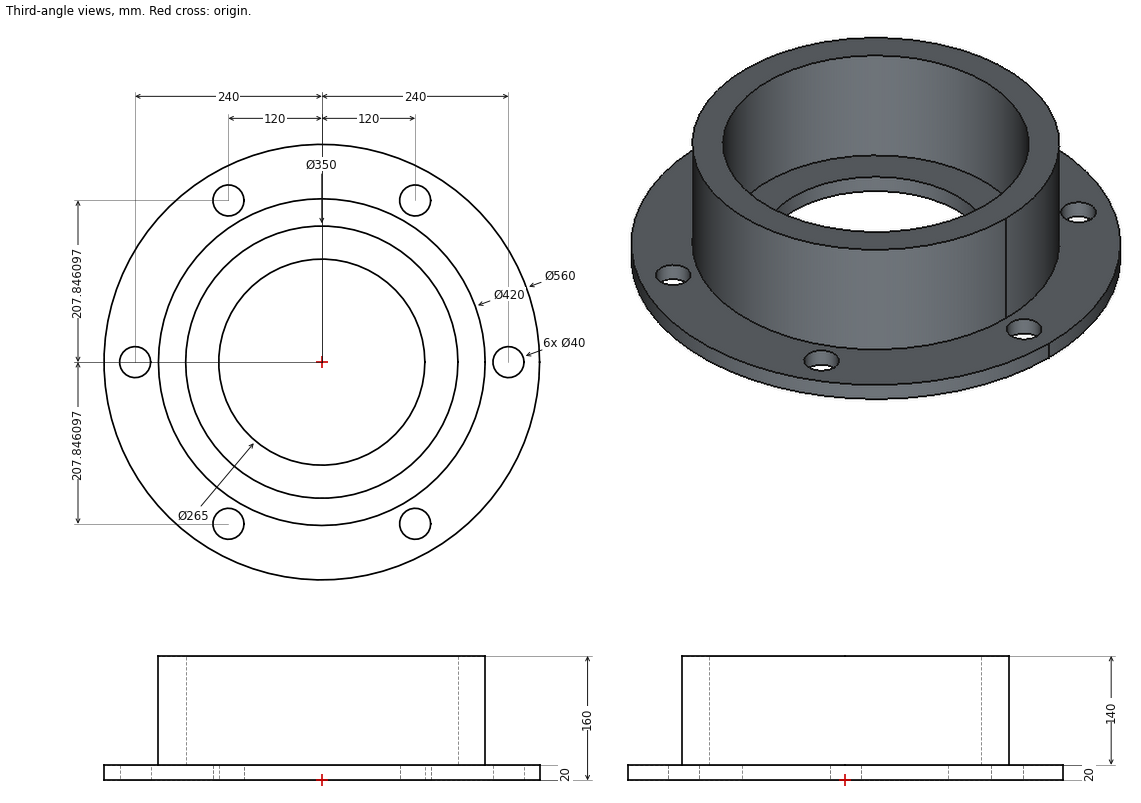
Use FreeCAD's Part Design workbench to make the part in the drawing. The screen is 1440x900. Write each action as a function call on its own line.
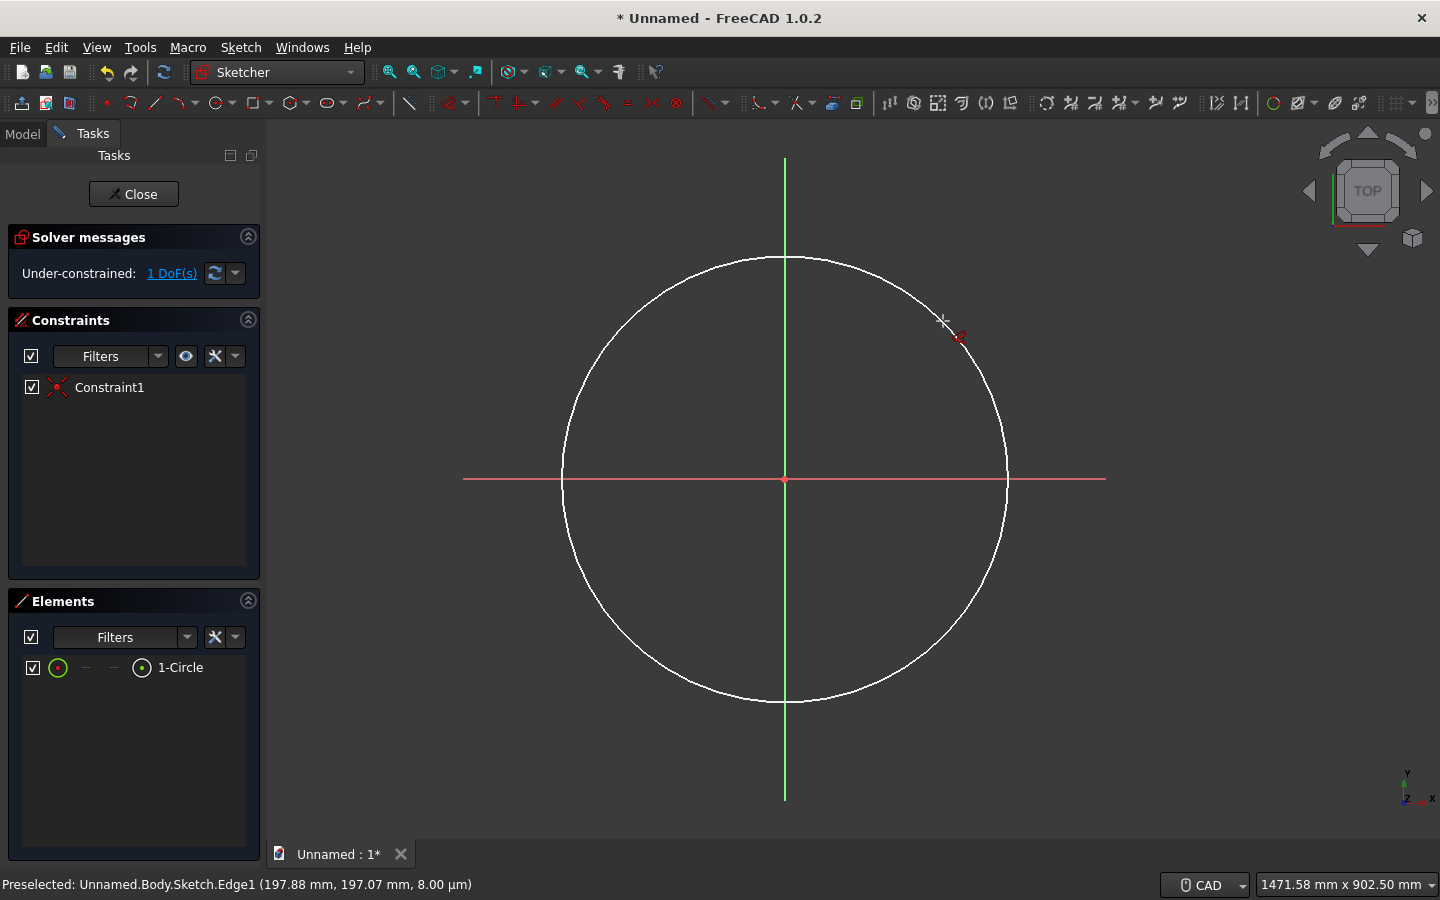
click(942, 321)
click(965, 298)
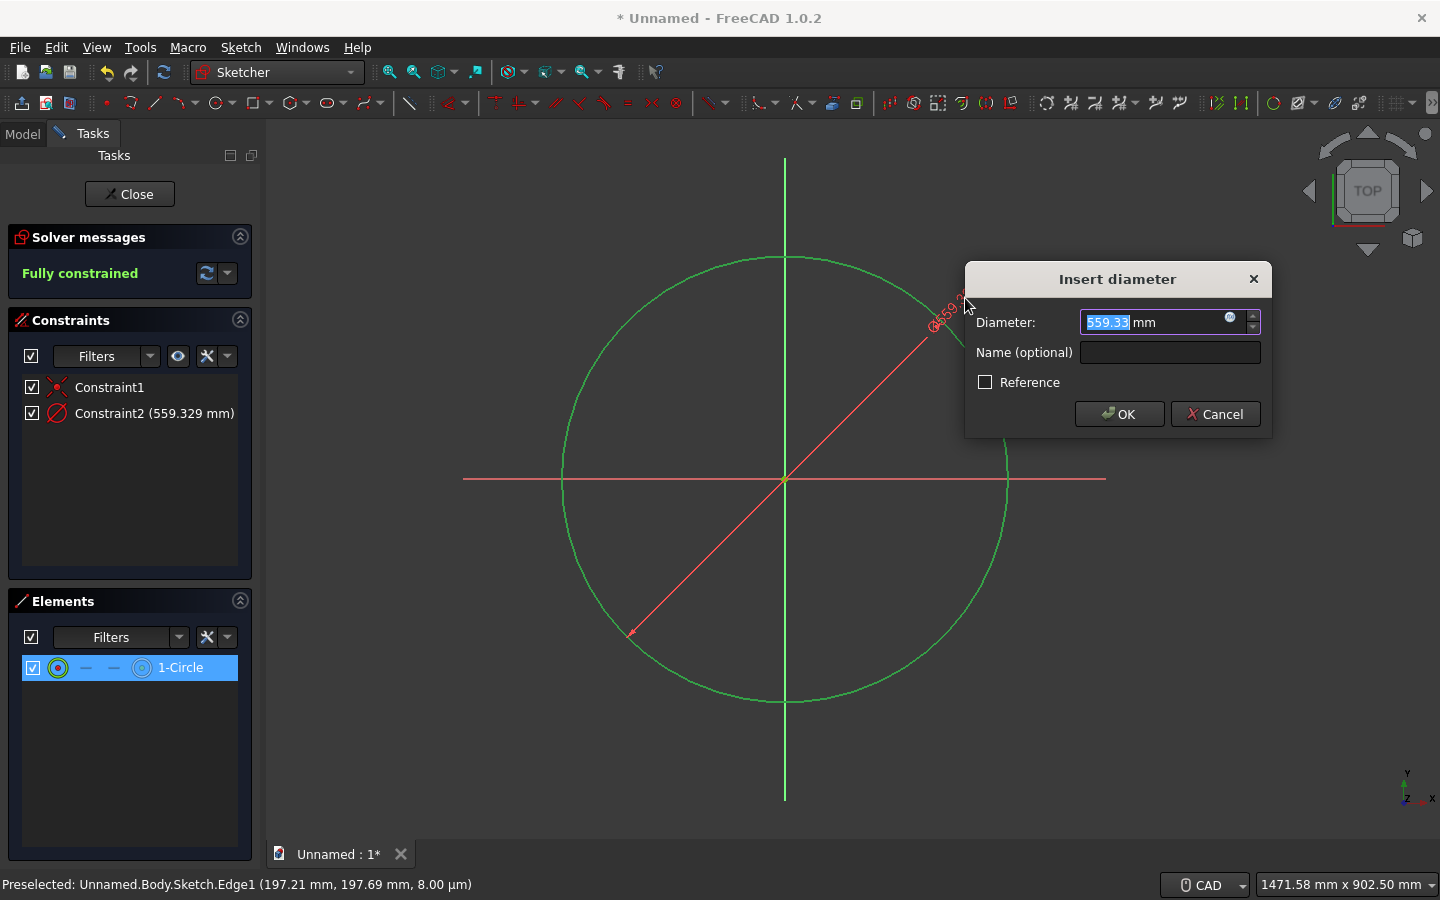
text(560)
key(Return)
key(Escape)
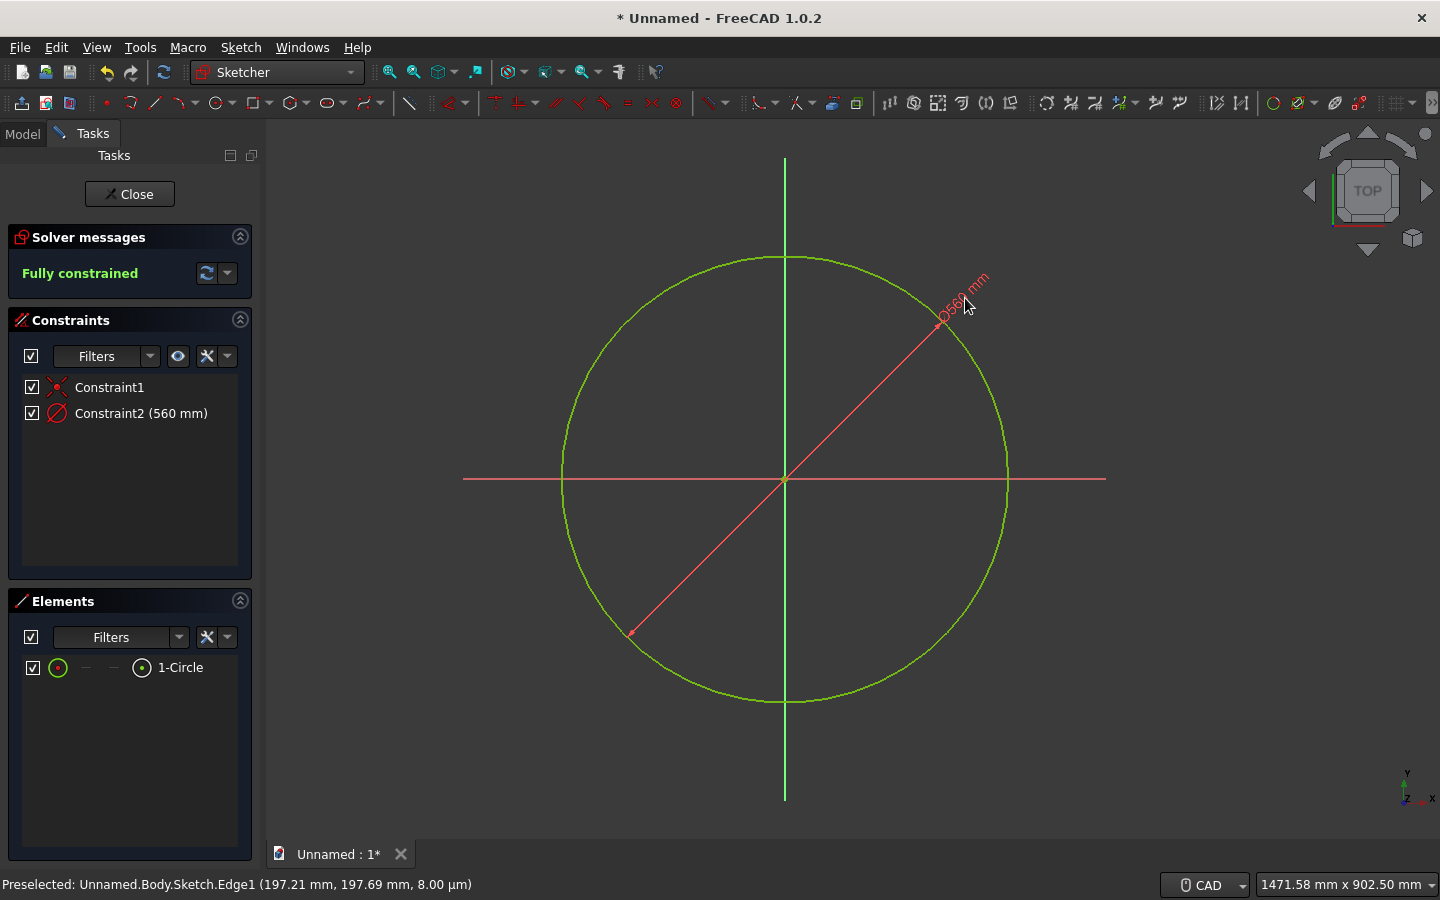
click(130, 194)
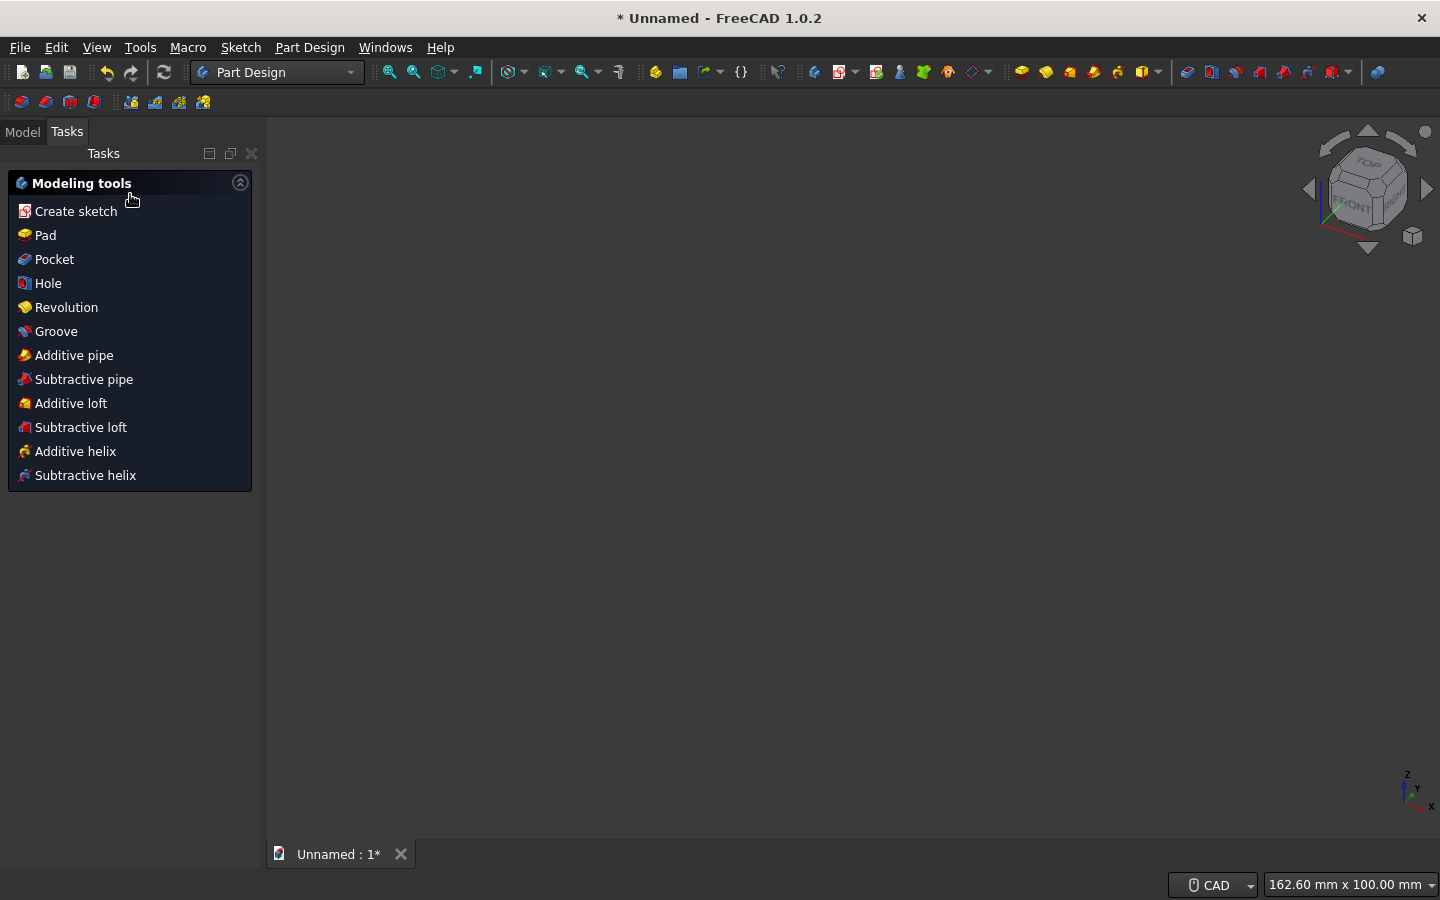
click(1022, 72)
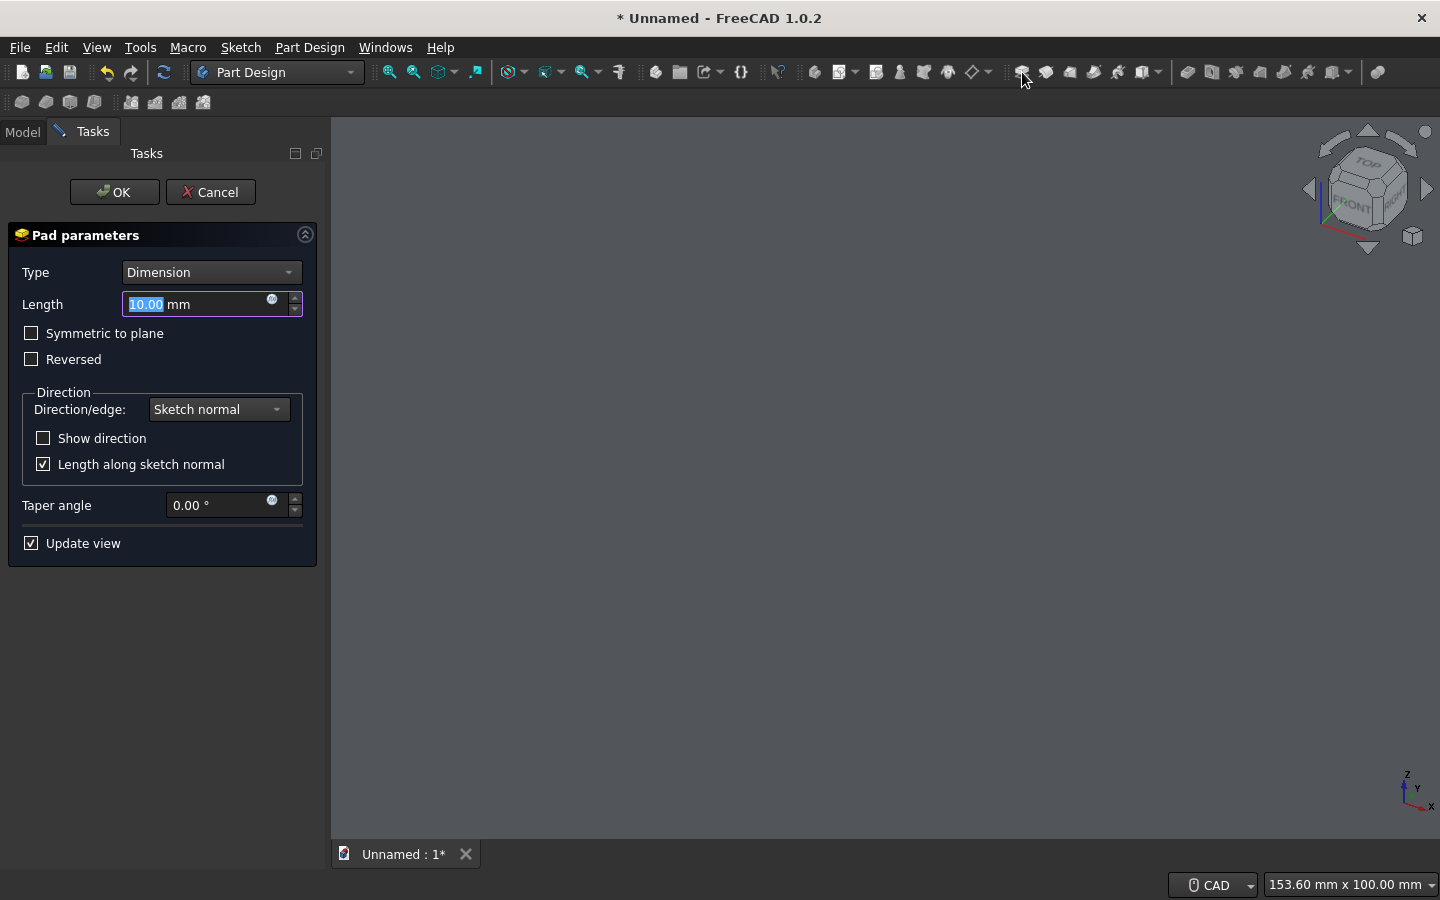
text(20)
key(Tab)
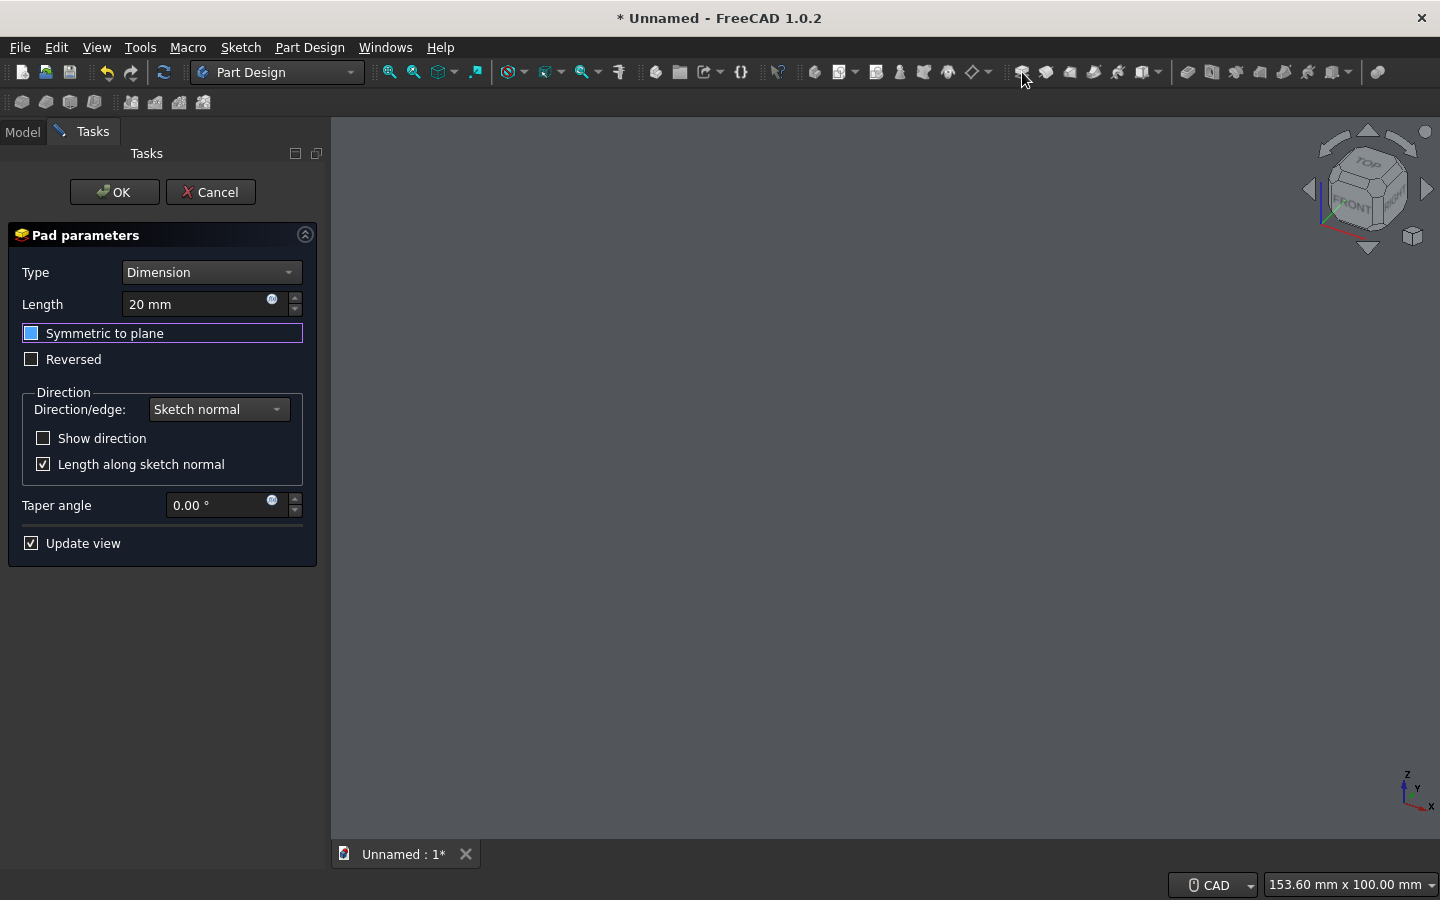
click(115, 192)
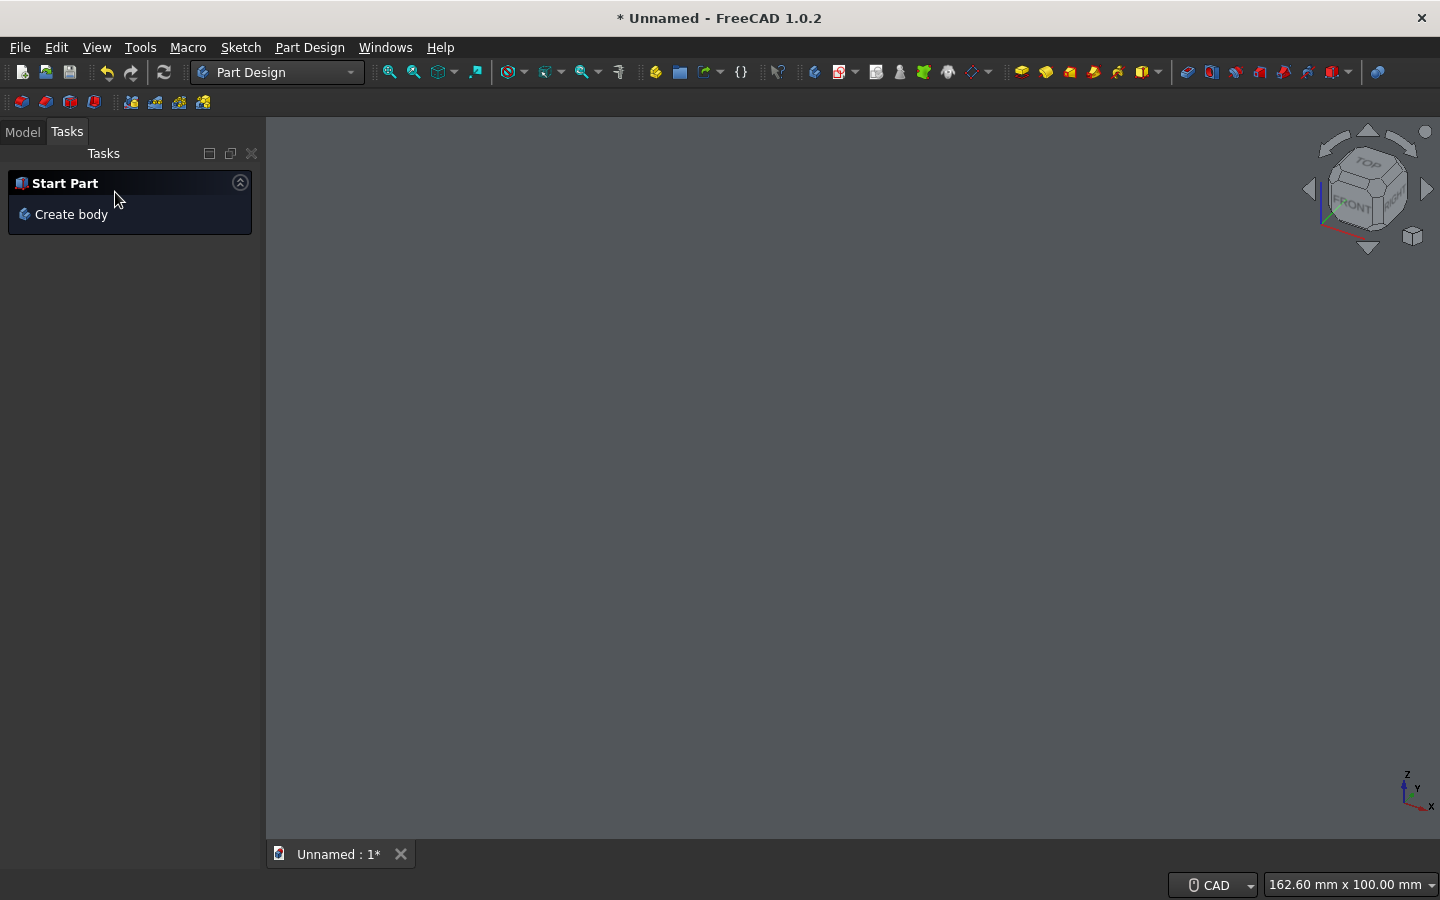
key(v)
key(f)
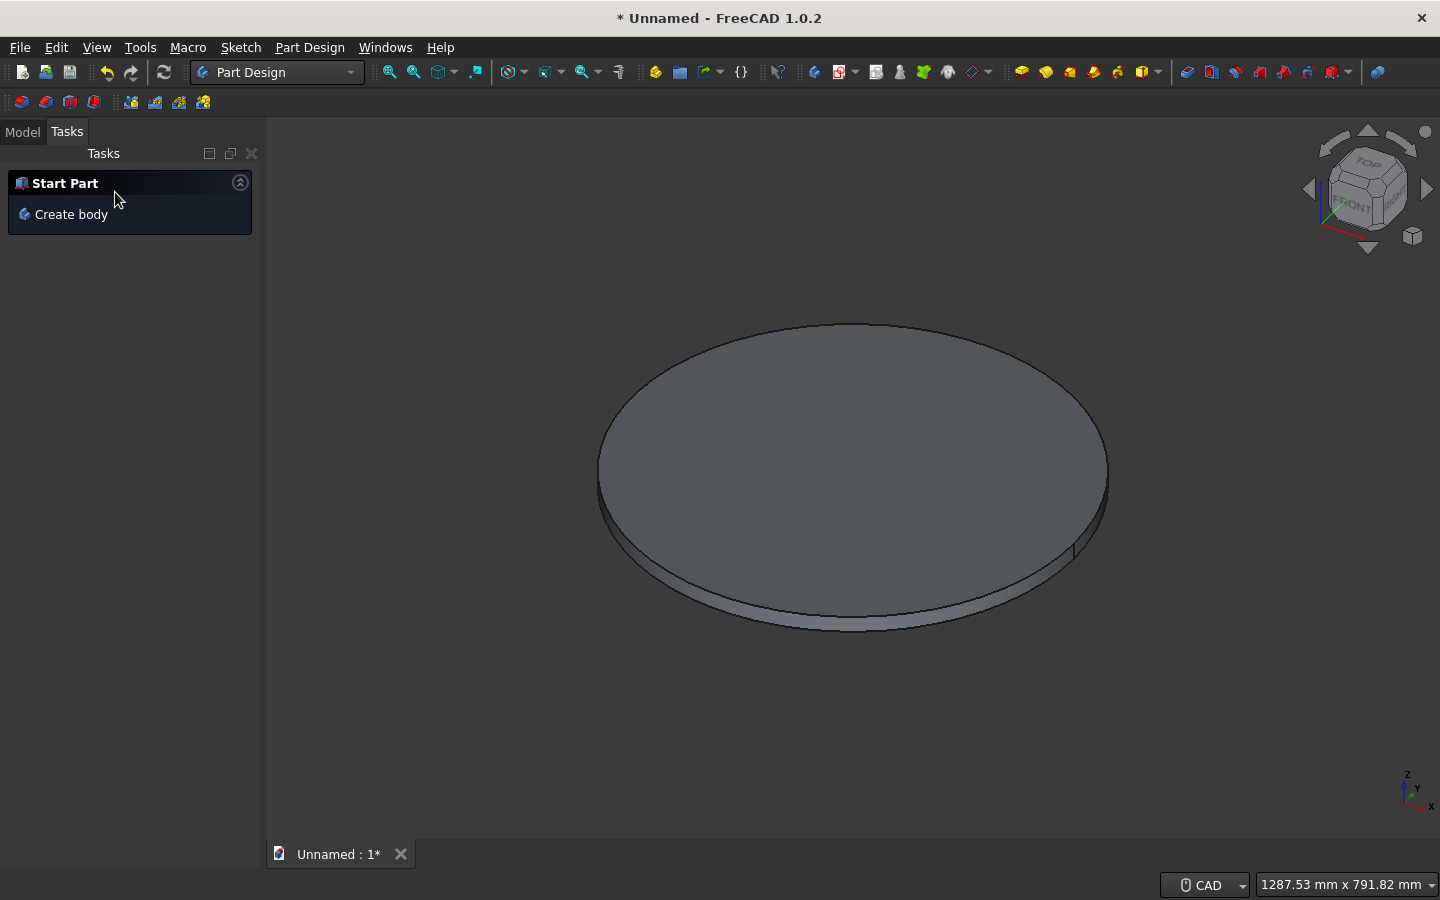
key(5)